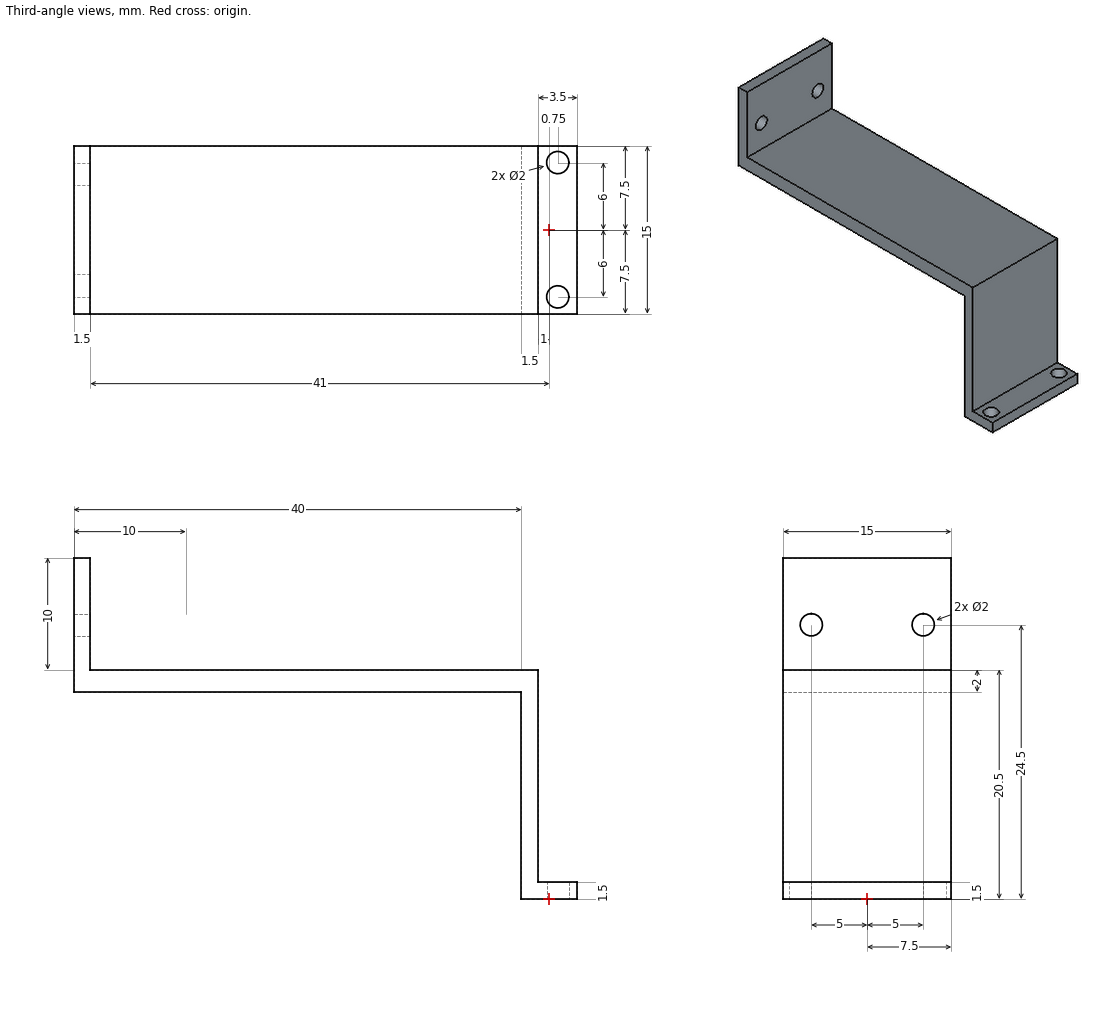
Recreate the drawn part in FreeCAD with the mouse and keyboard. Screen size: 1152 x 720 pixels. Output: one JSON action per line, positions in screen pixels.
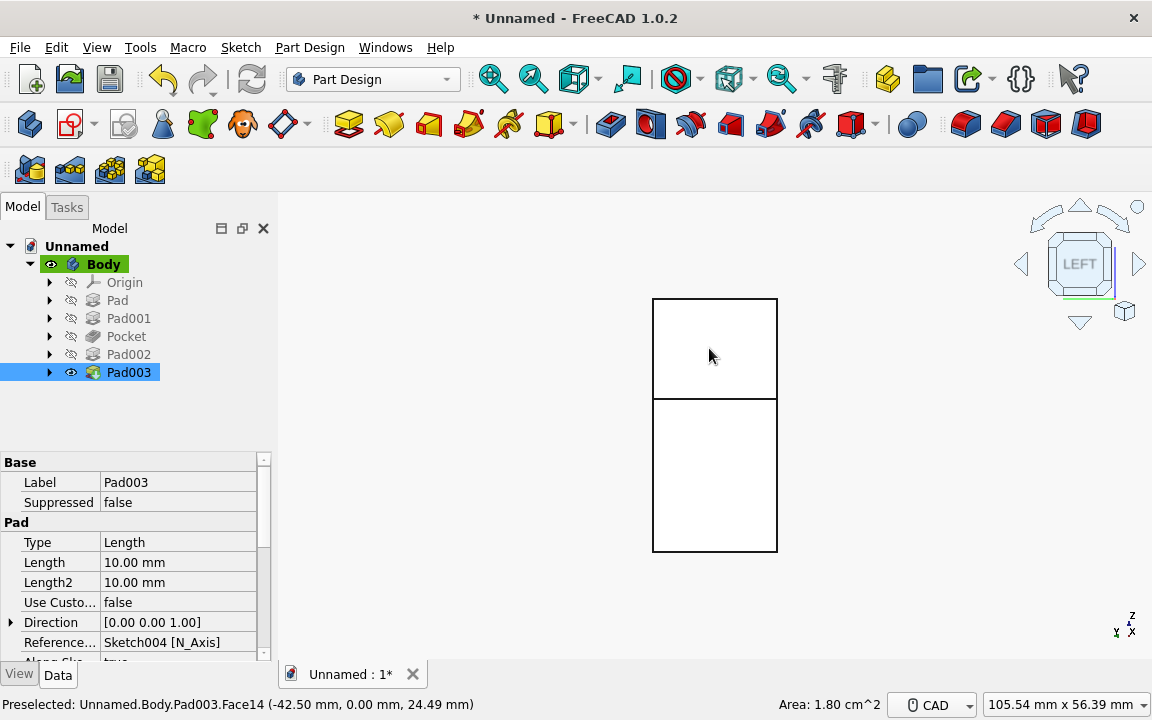
{"action": "left_click", "coordinate": [70, 124]}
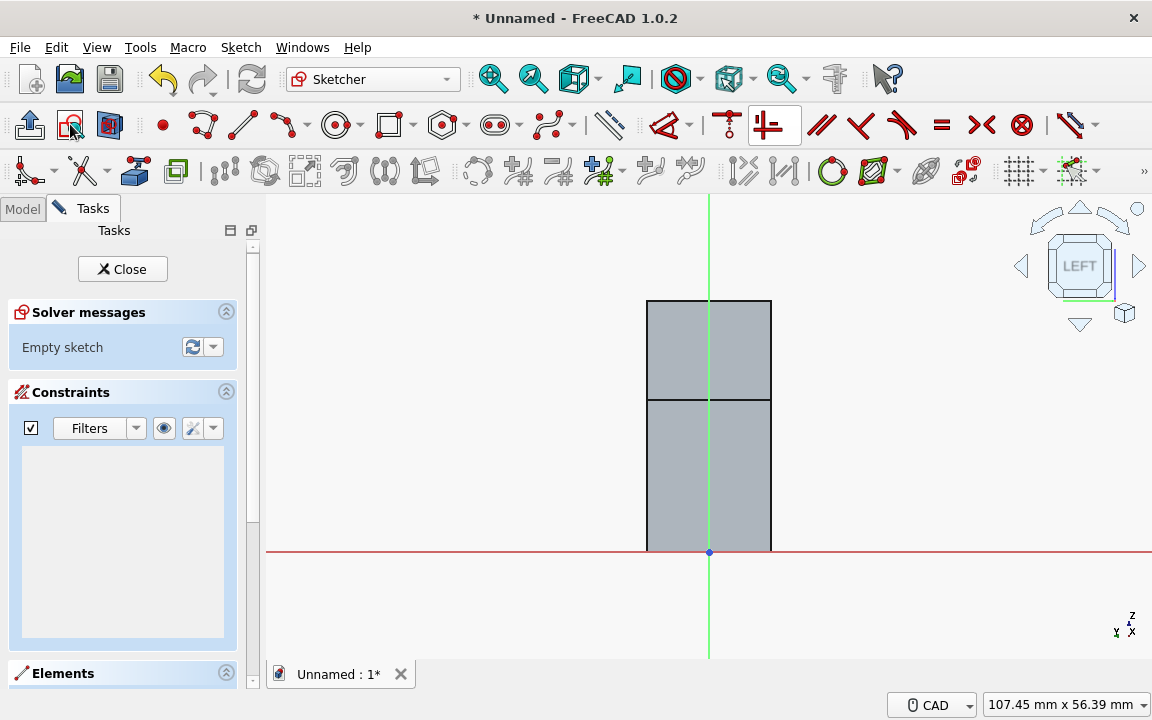
{"action": "scroll", "coordinate": [848, 489], "scroll_direction": "up", "scroll_amount": 2}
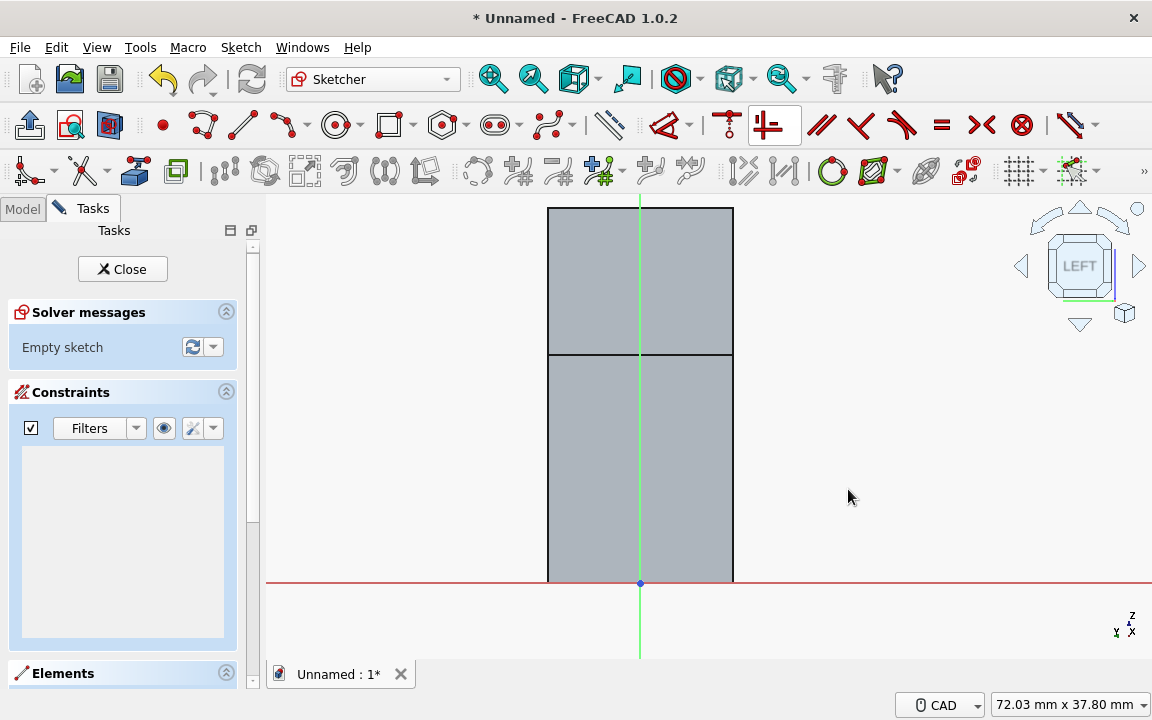
{"action": "left_click", "coordinate": [336, 126]}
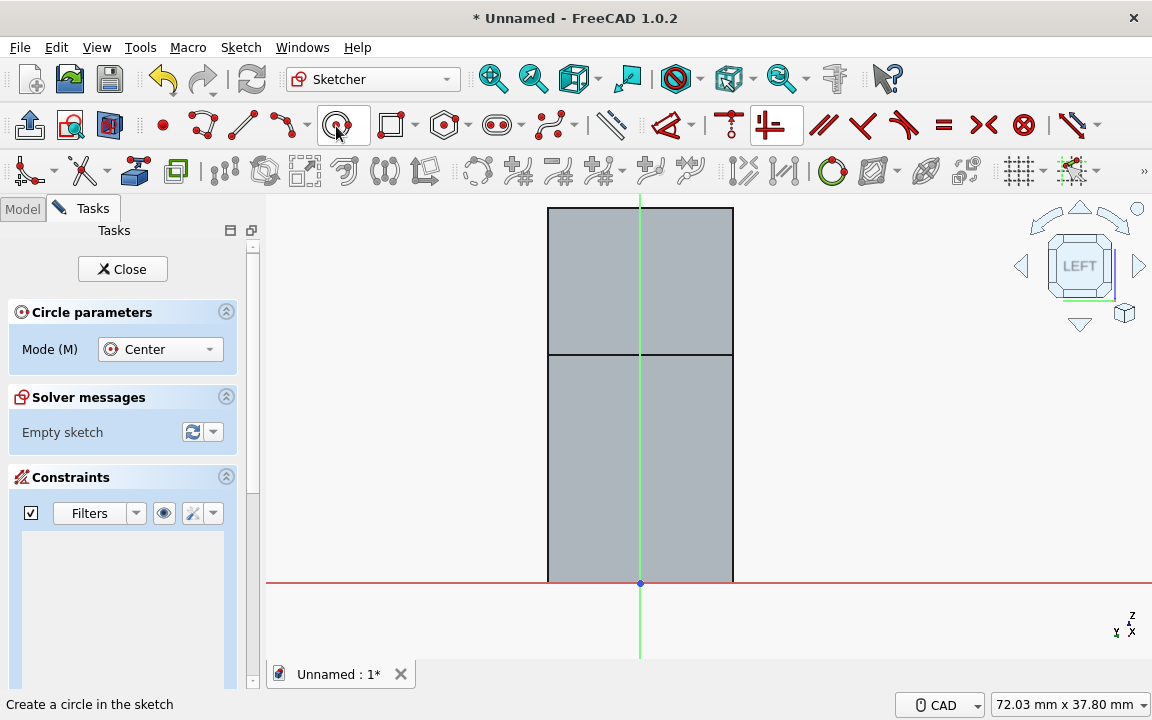
{"action": "scroll", "coordinate": [579, 282], "scroll_direction": "up", "scroll_amount": 4}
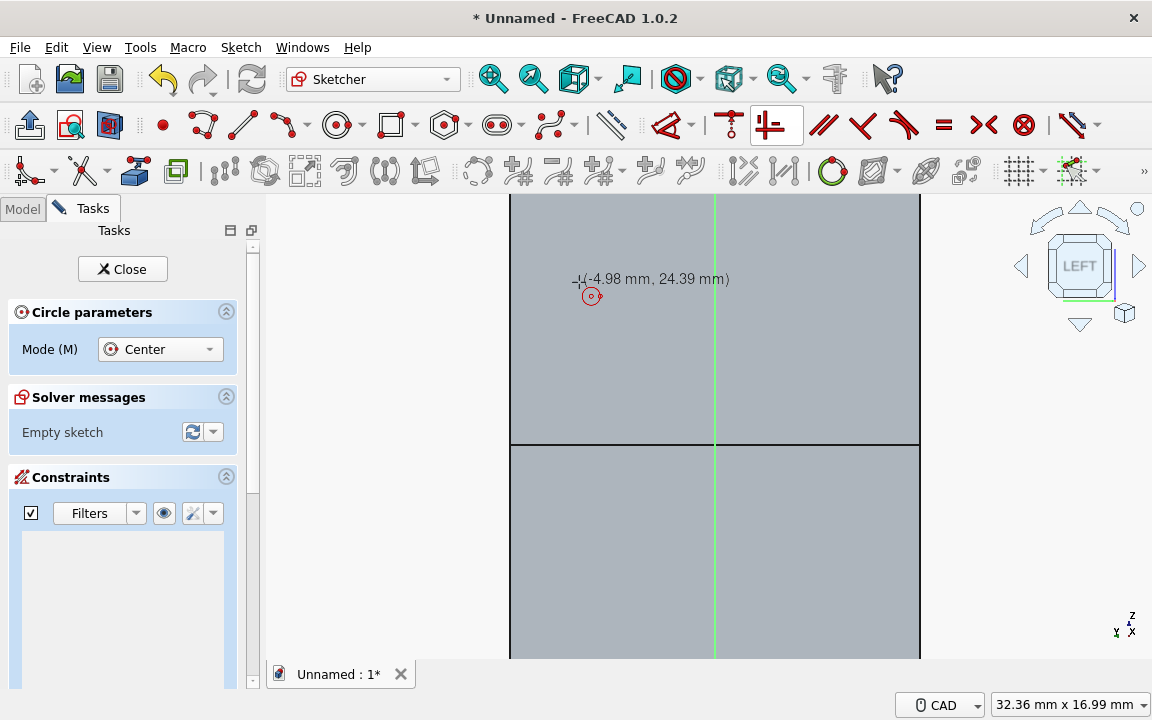
{"action": "left_click", "coordinate": [578, 281]}
{"action": "left_click", "coordinate": [597, 262]}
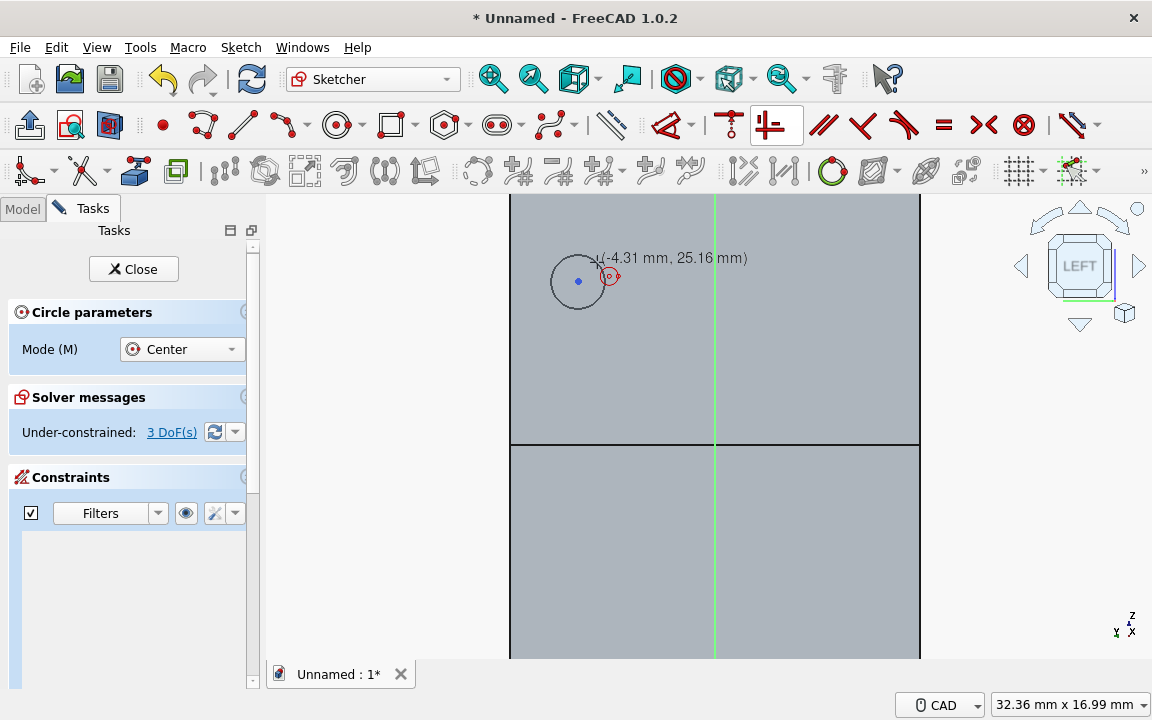
{"action": "left_click", "coordinate": [852, 281]}
{"action": "left_click", "coordinate": [871, 262]}
{"action": "key", "text": "Escape"}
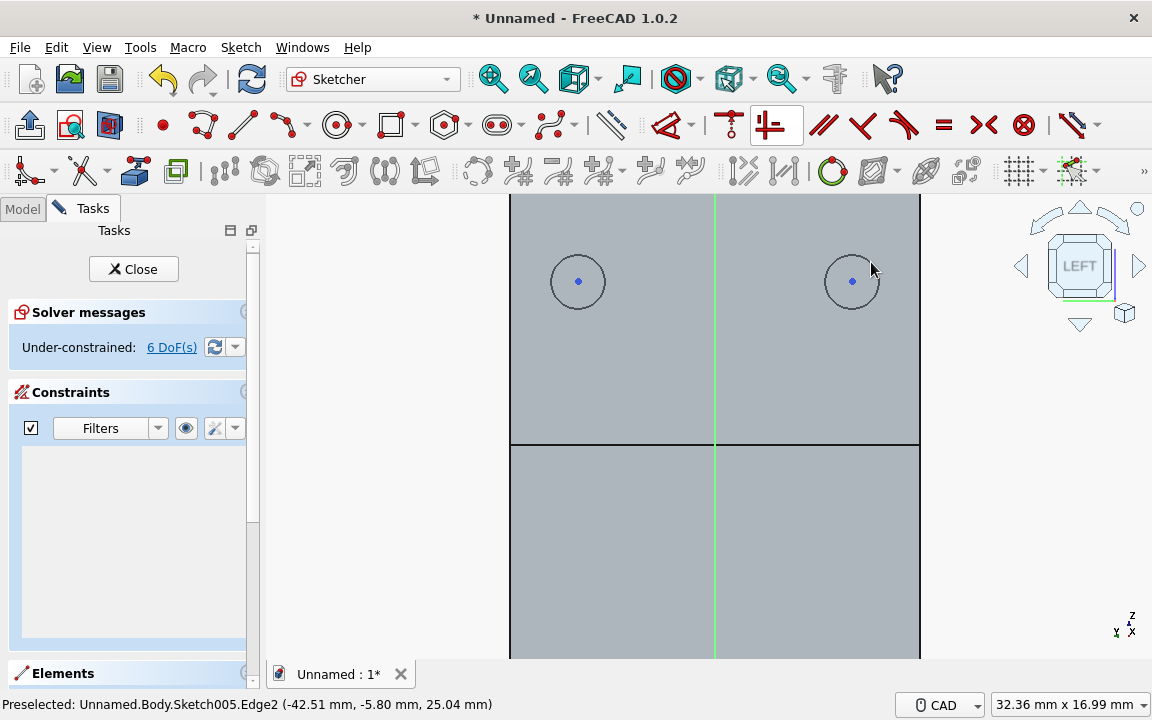
{"action": "left_click", "coordinate": [597, 263]}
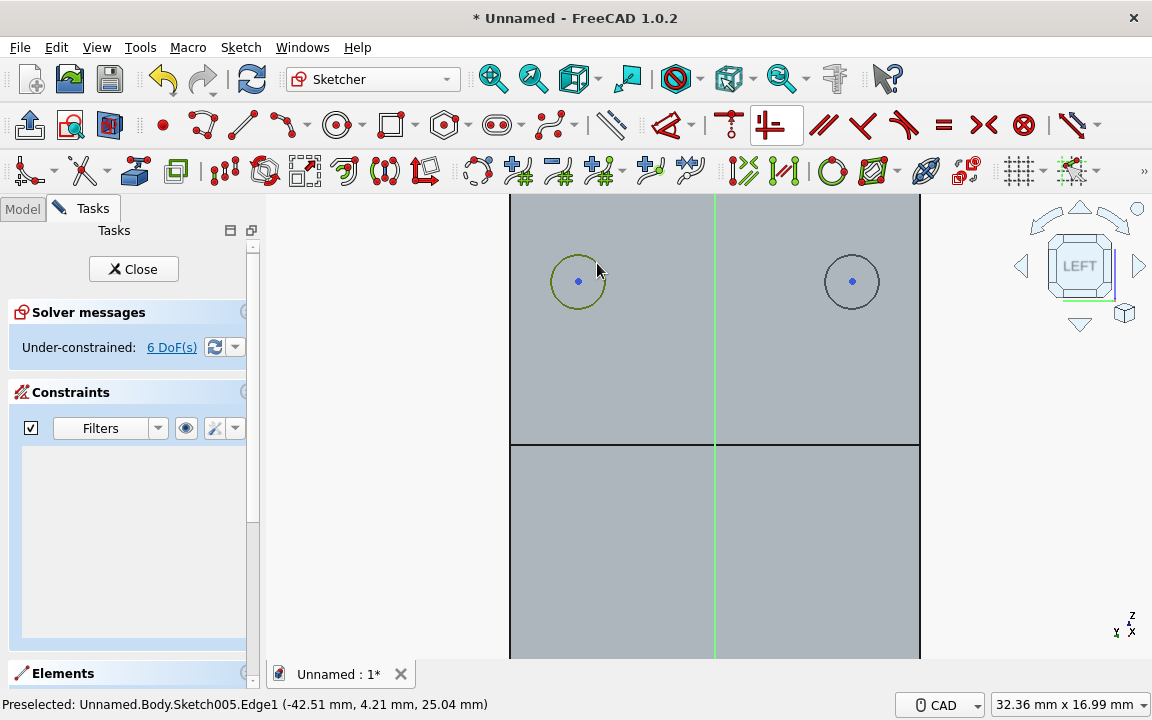
{"action": "left_click", "coordinate": [871, 263]}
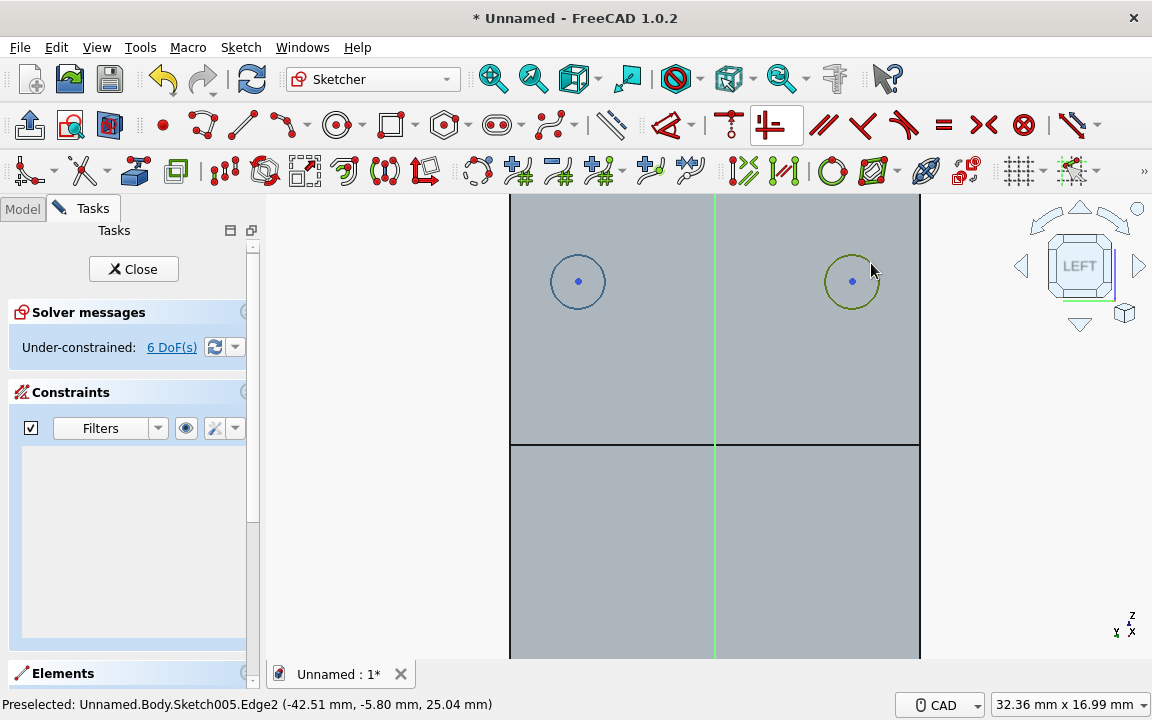
{"action": "left_click", "coordinate": [944, 126]}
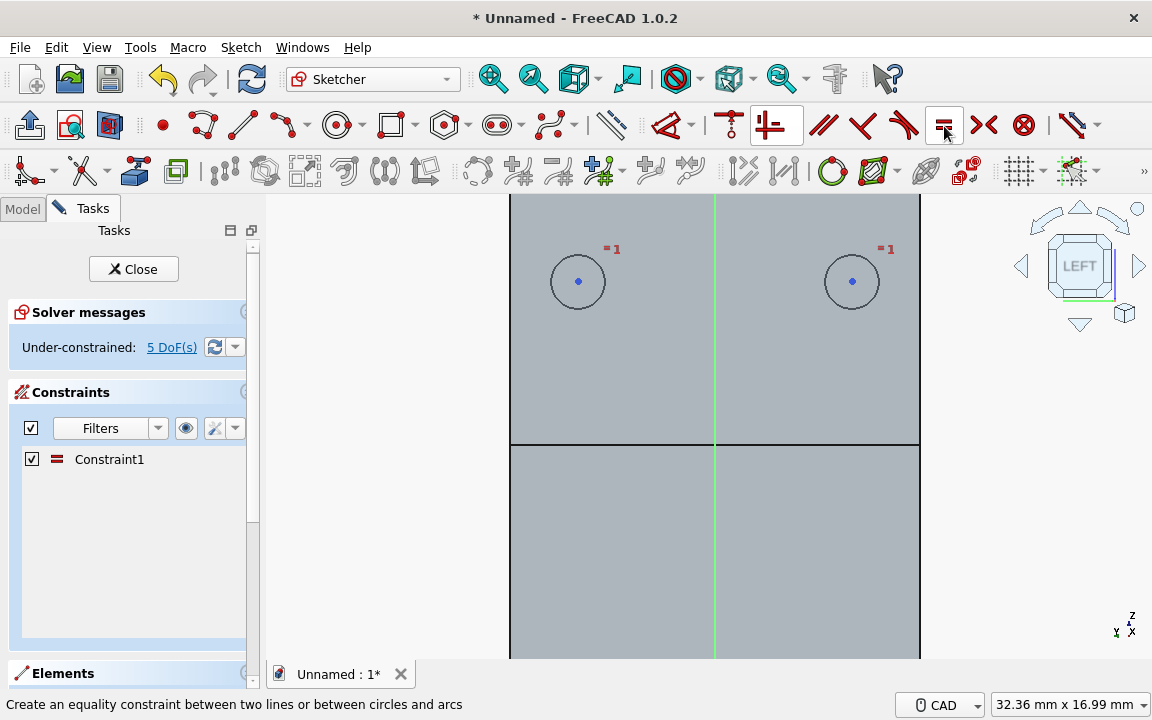
{"action": "left_click", "coordinate": [578, 282]}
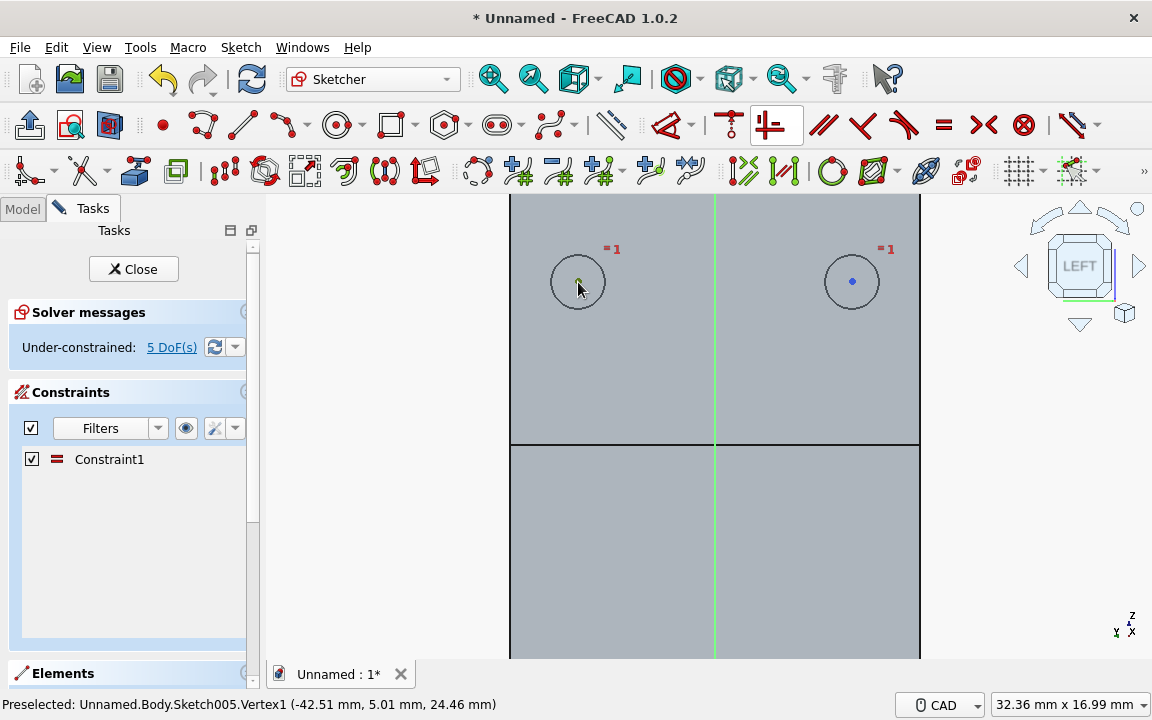
{"action": "left_click", "coordinate": [852, 282]}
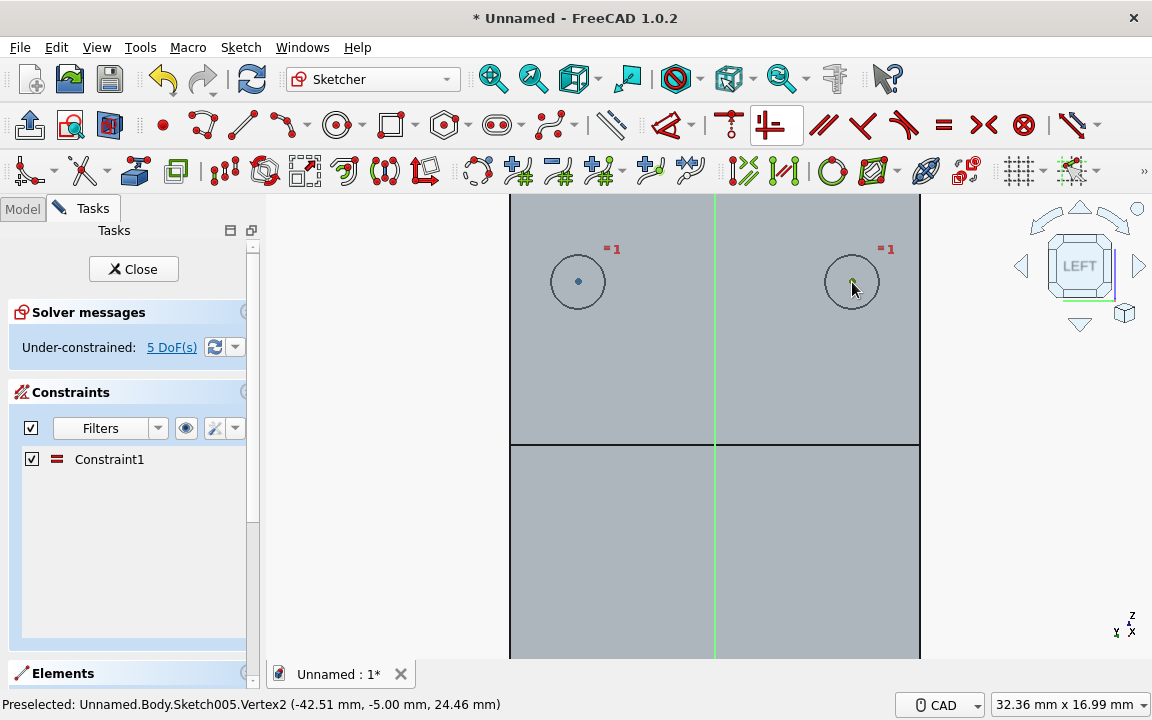
{"action": "left_click", "coordinate": [798, 126]}